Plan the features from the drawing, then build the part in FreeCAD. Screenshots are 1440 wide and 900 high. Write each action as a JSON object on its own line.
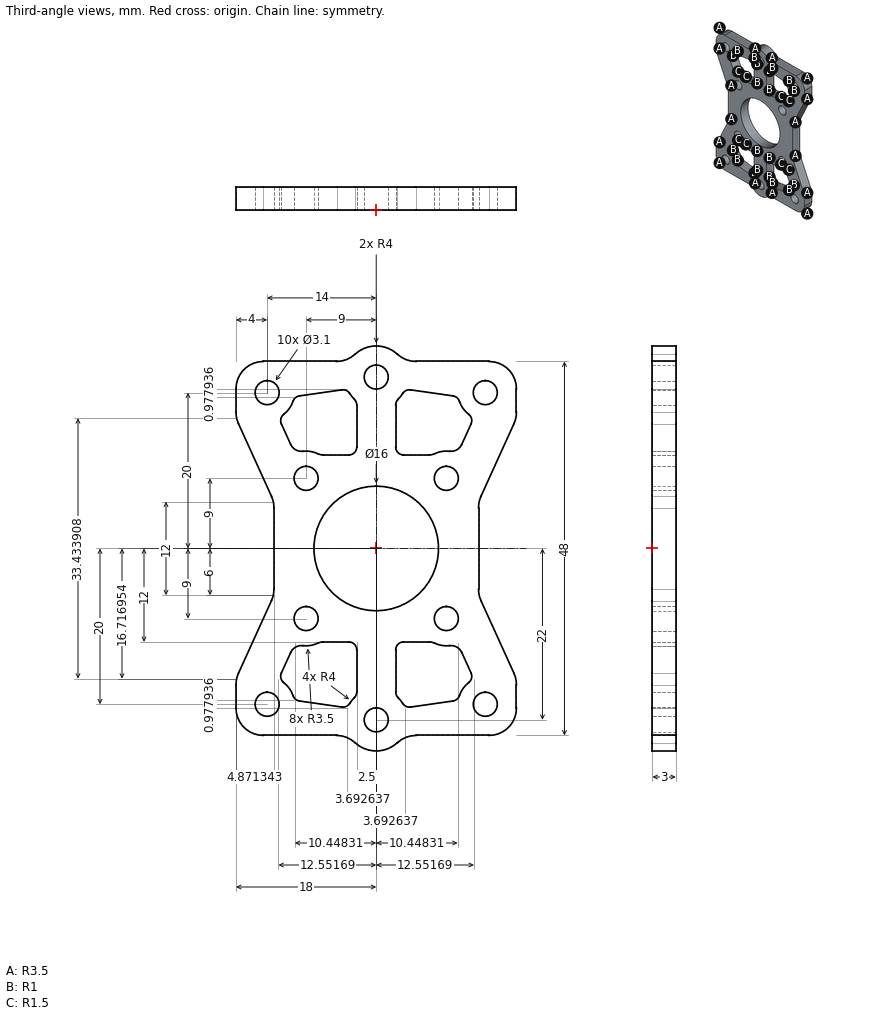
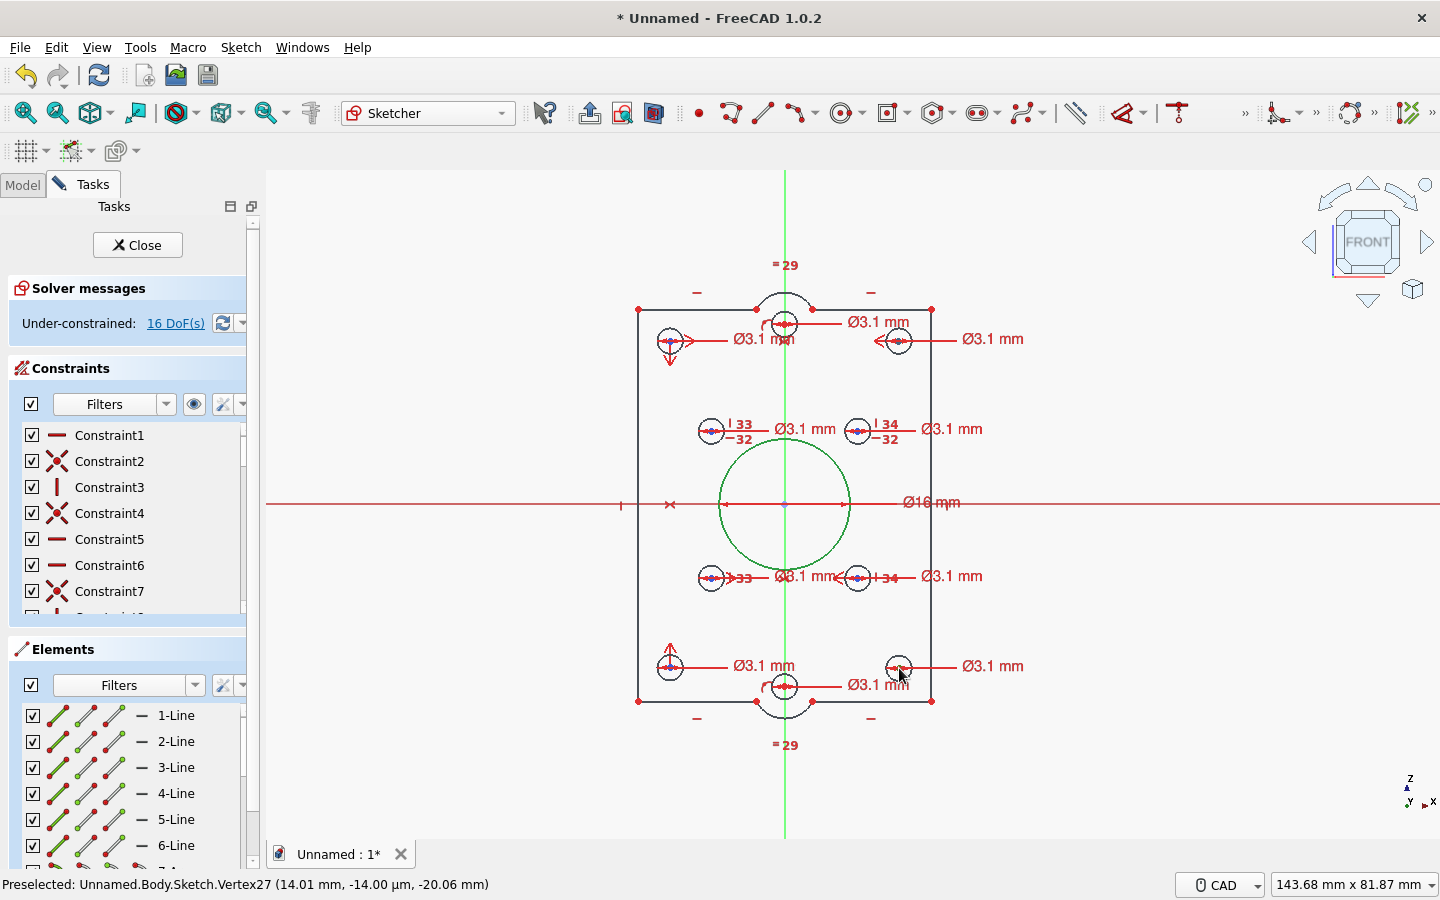
{"action": "left_click", "coordinate": [364, 504]}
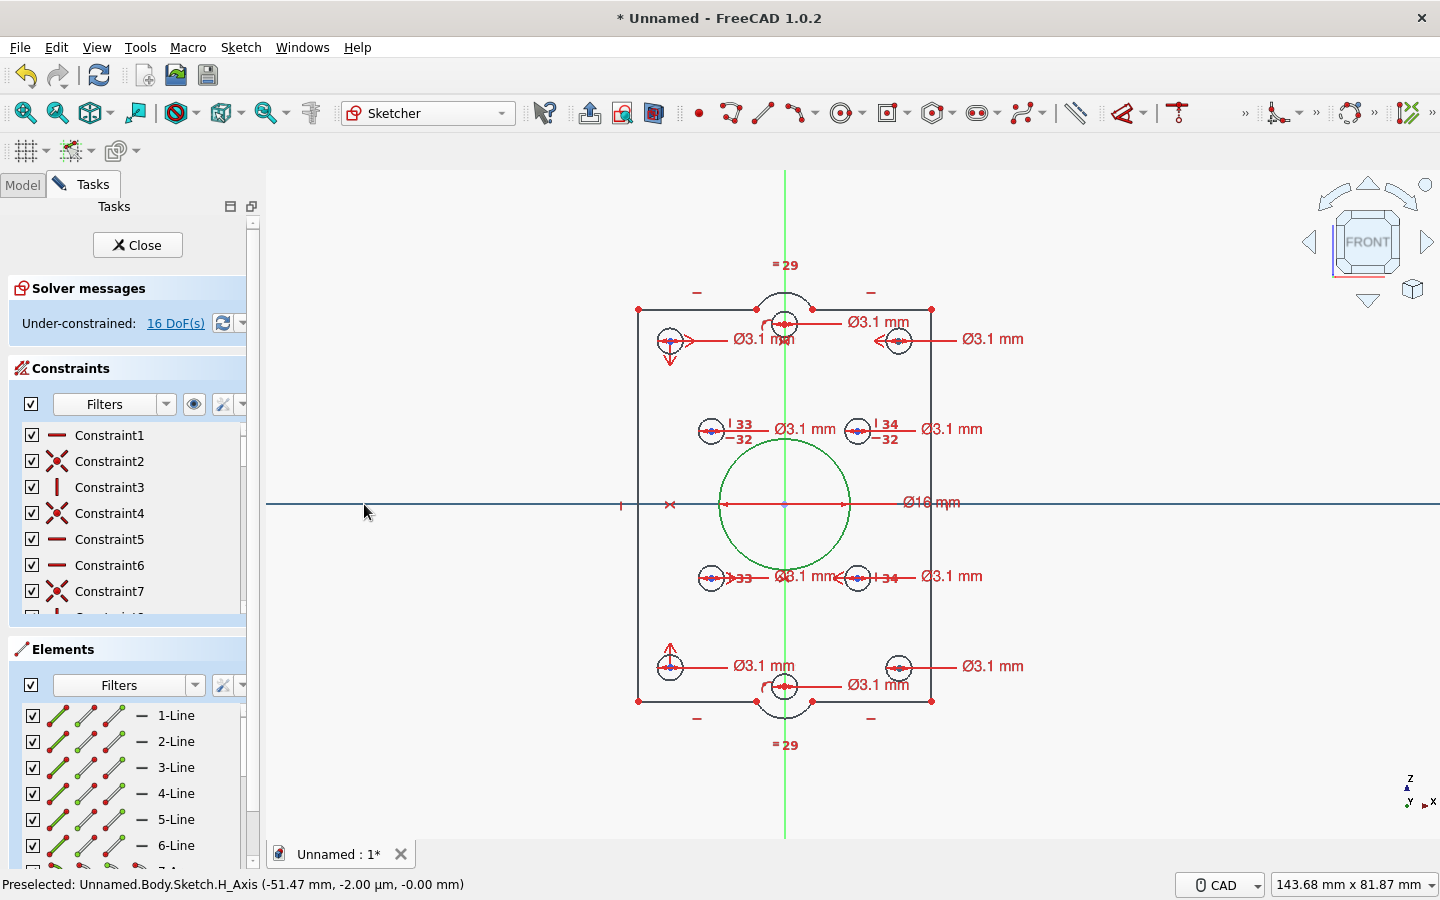
{"action": "key", "text": "s"}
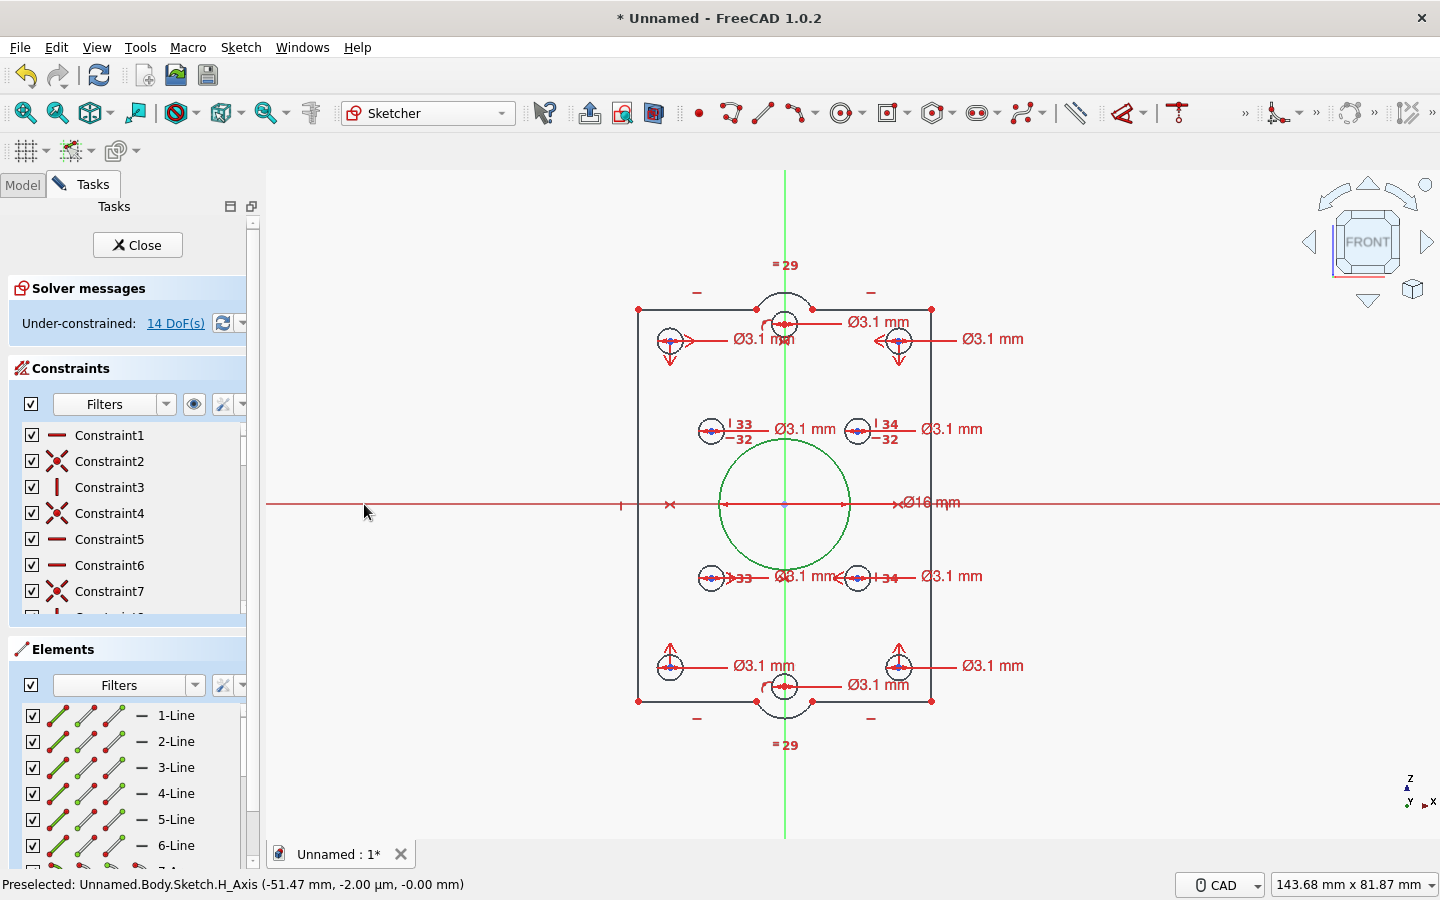
{"action": "left_click", "coordinate": [813, 310]}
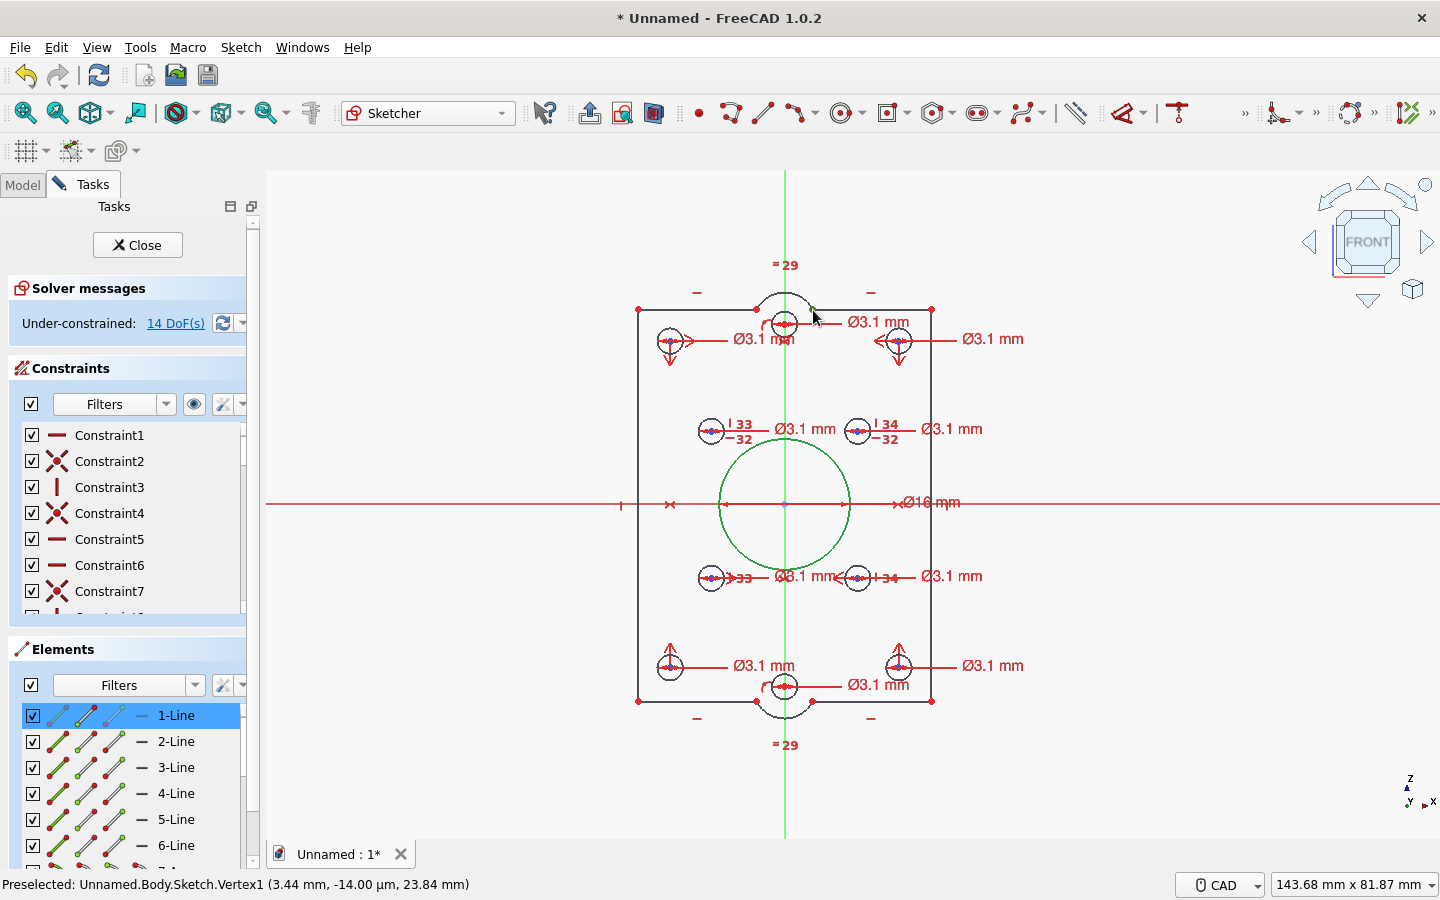
{"action": "left_click", "coordinate": [813, 702]}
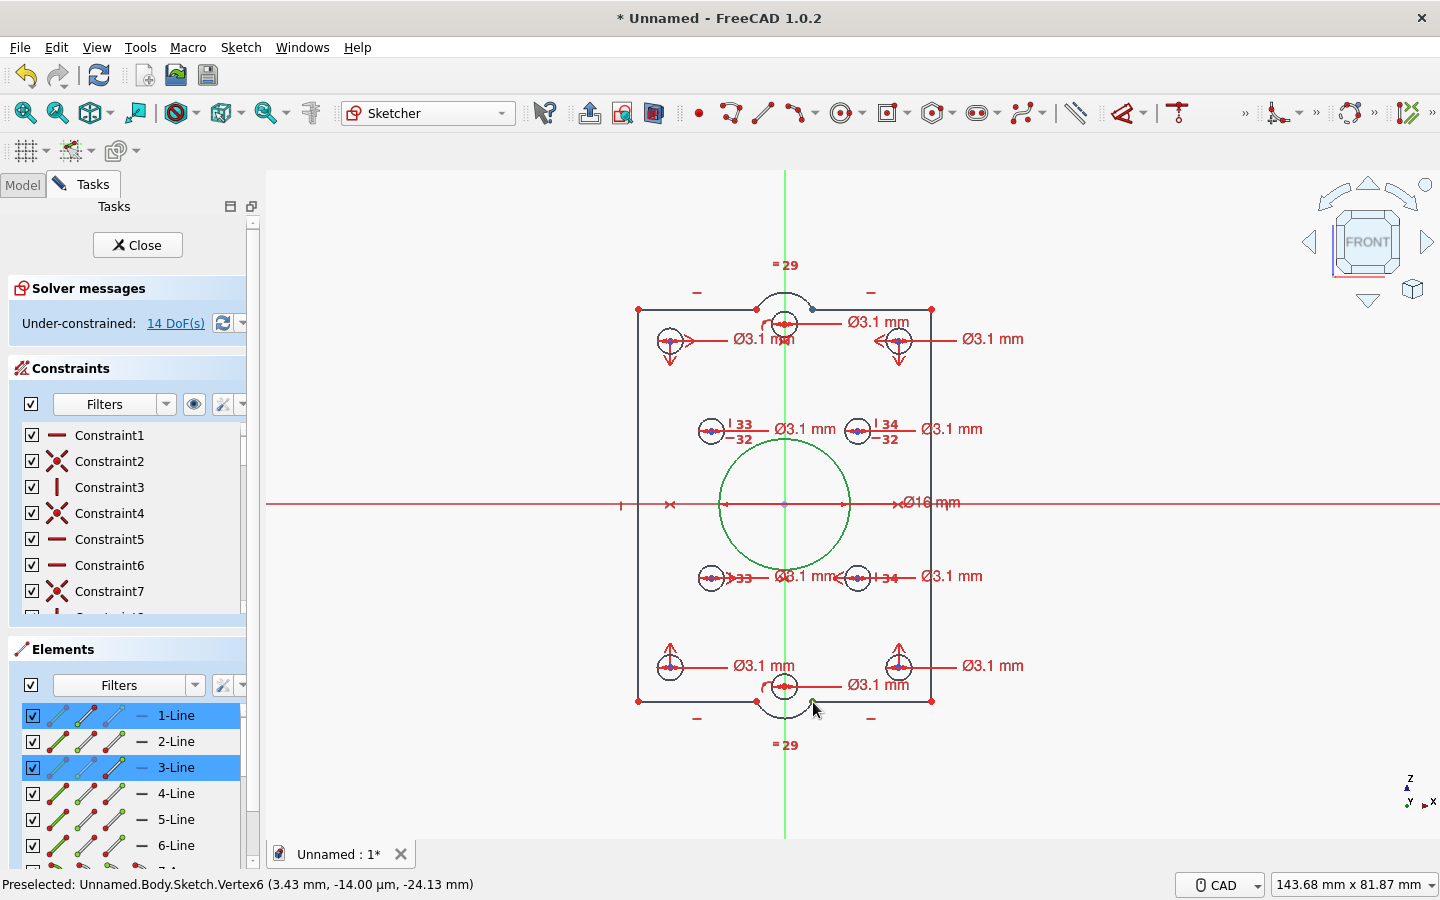
{"action": "left_click", "coordinate": [364, 504]}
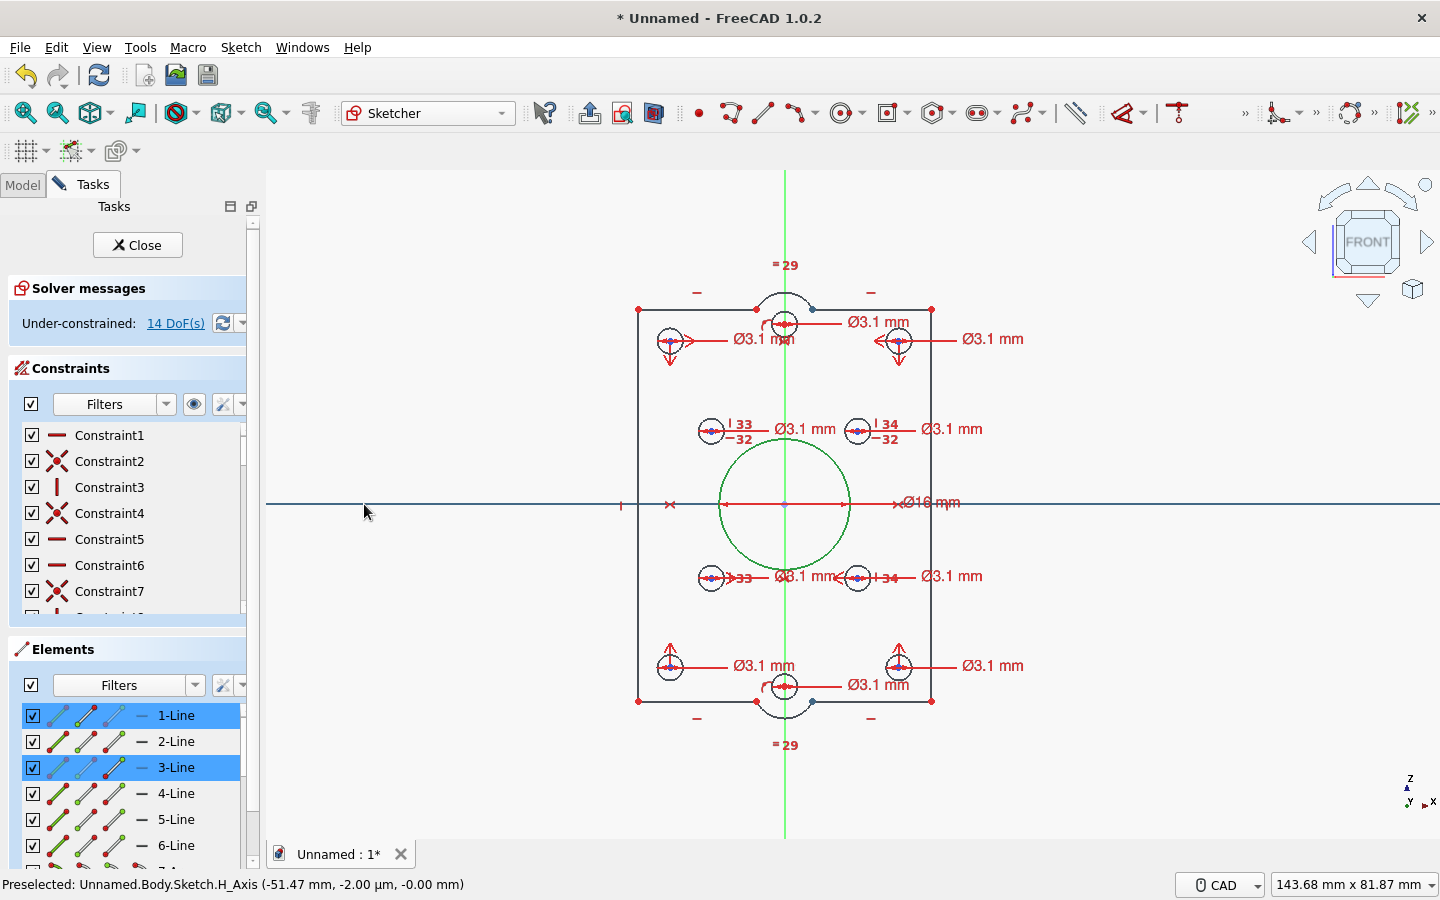
{"action": "key", "text": "s"}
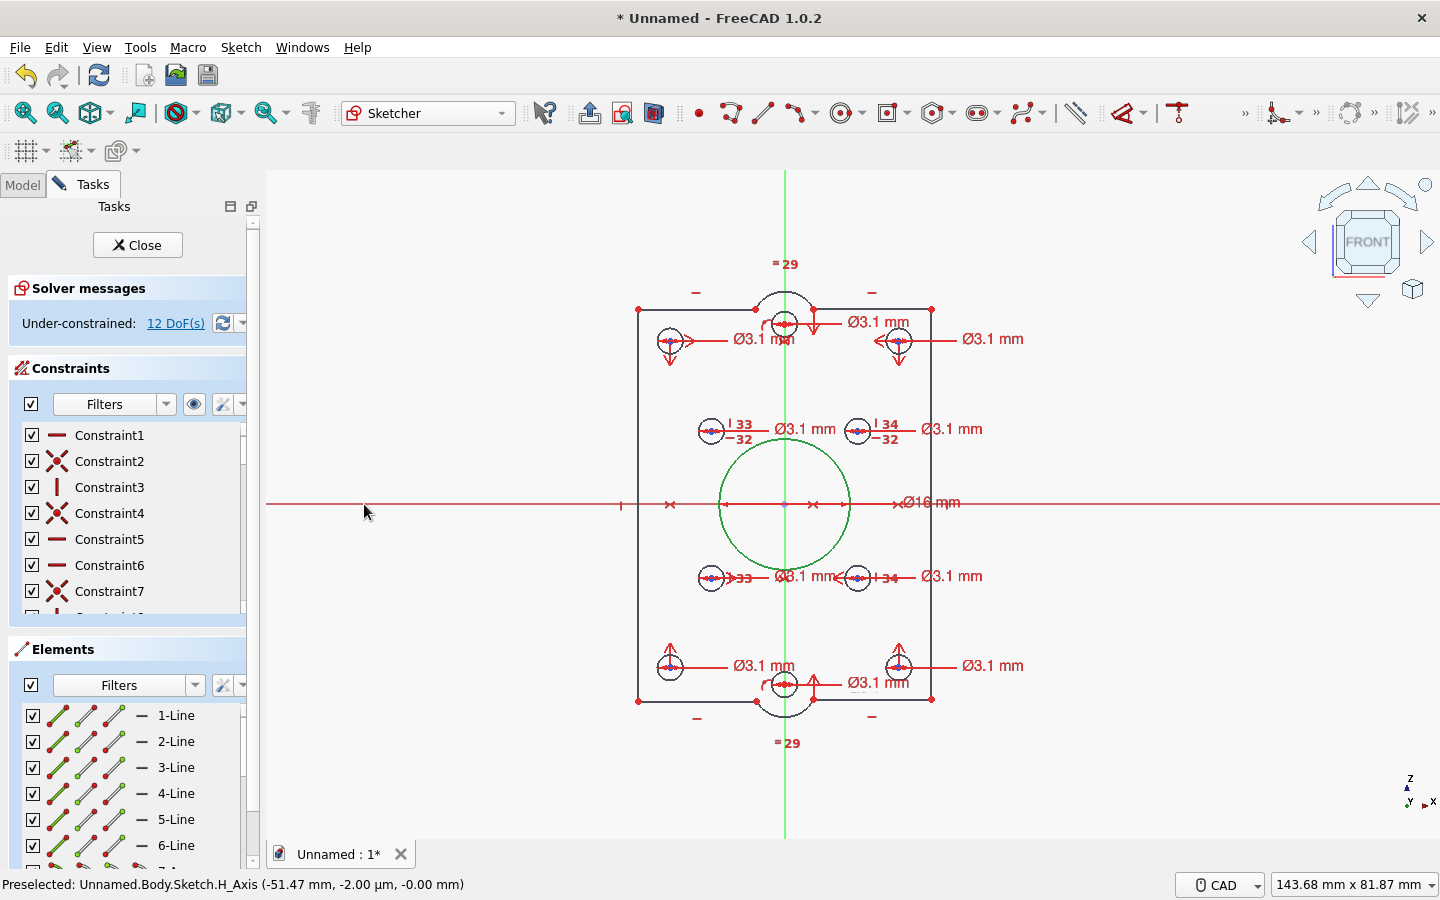
{"action": "left_click", "coordinate": [931, 700]}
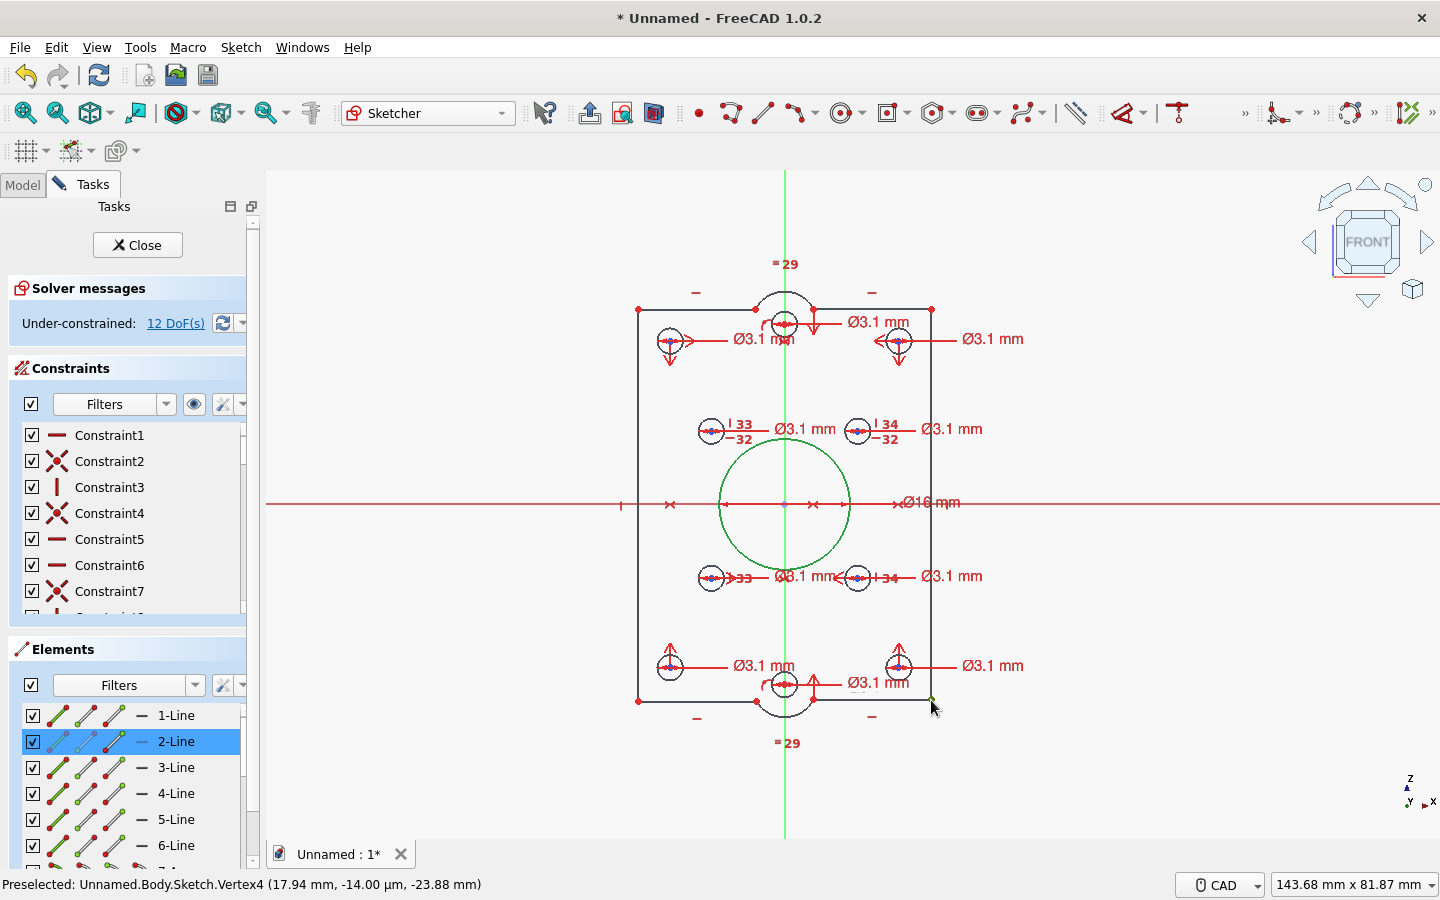
{"action": "left_click", "coordinate": [638, 702]}